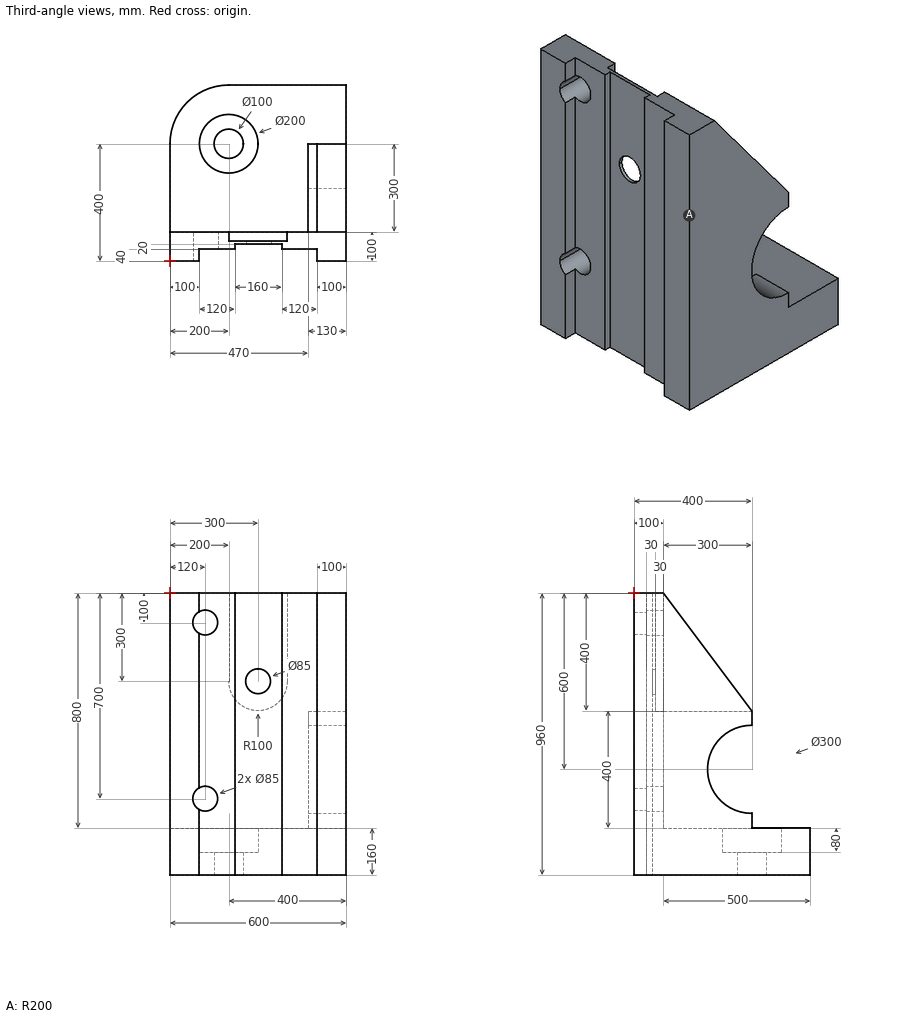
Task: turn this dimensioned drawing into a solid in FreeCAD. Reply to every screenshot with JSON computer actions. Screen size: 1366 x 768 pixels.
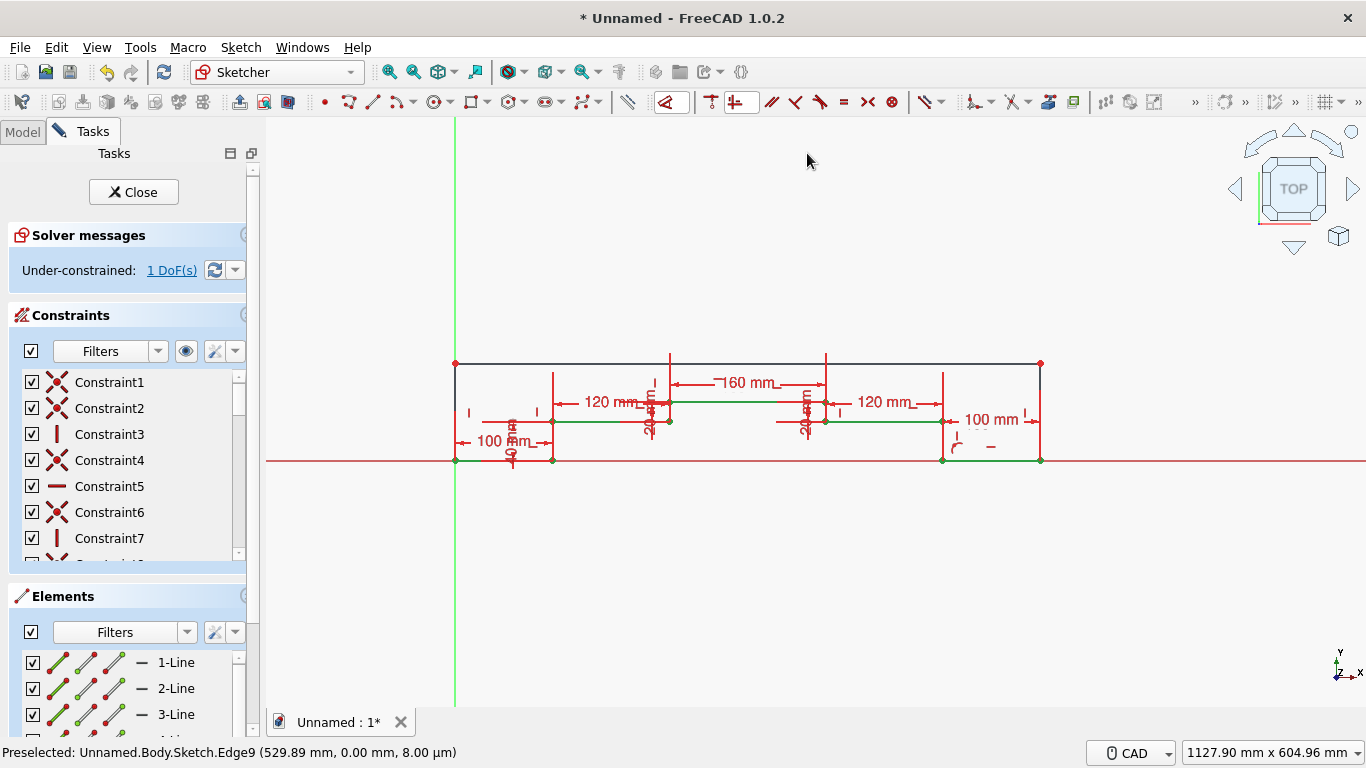
{"action": "left_click", "coordinate": [1040, 432]}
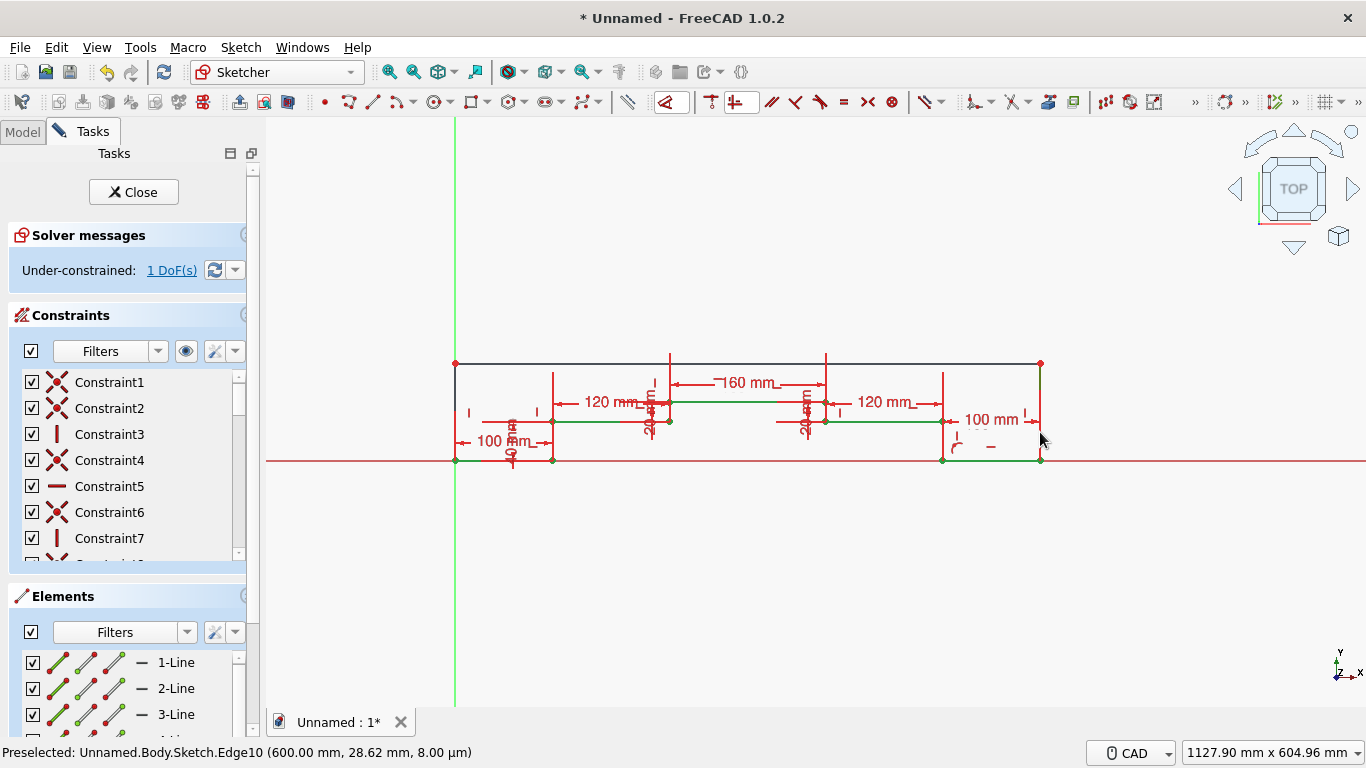
{"action": "key", "text": "i"}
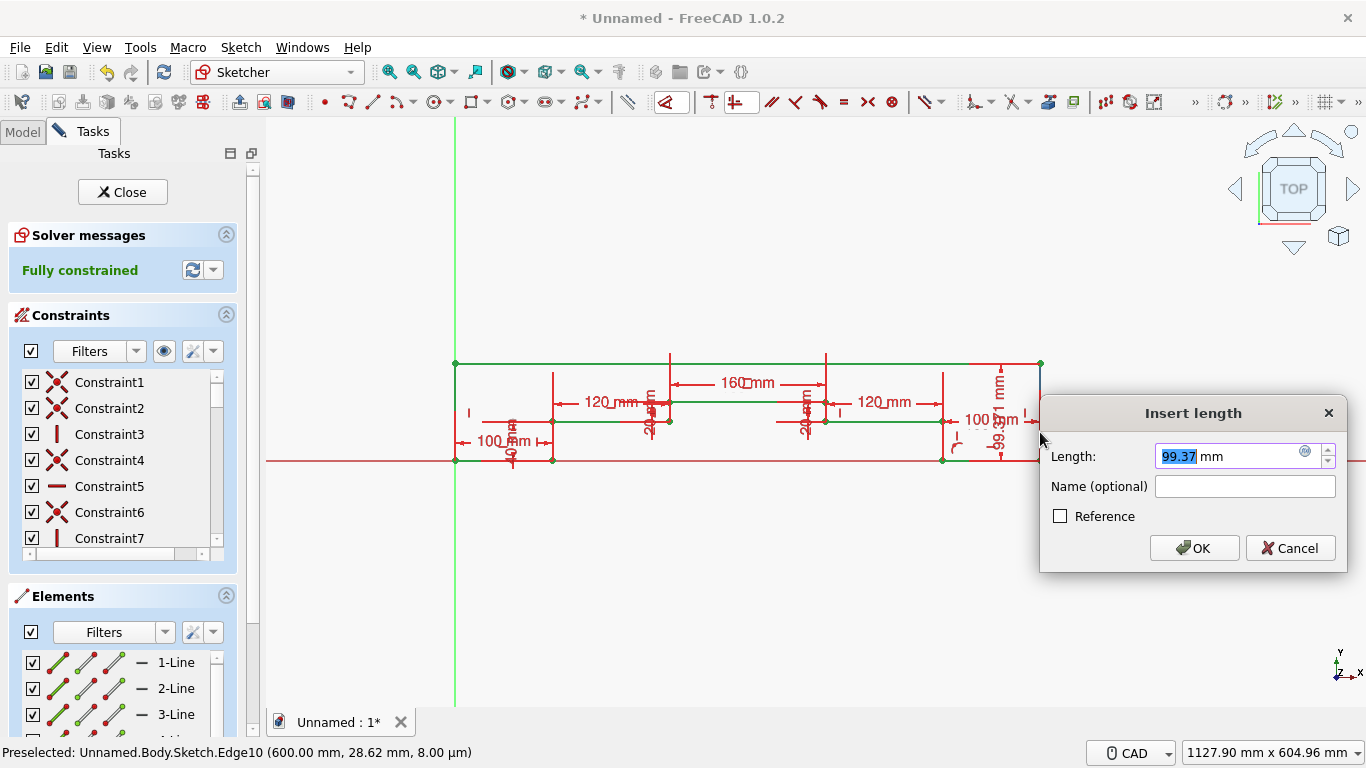
{"action": "type", "text": "100"}
{"action": "key", "text": "Return"}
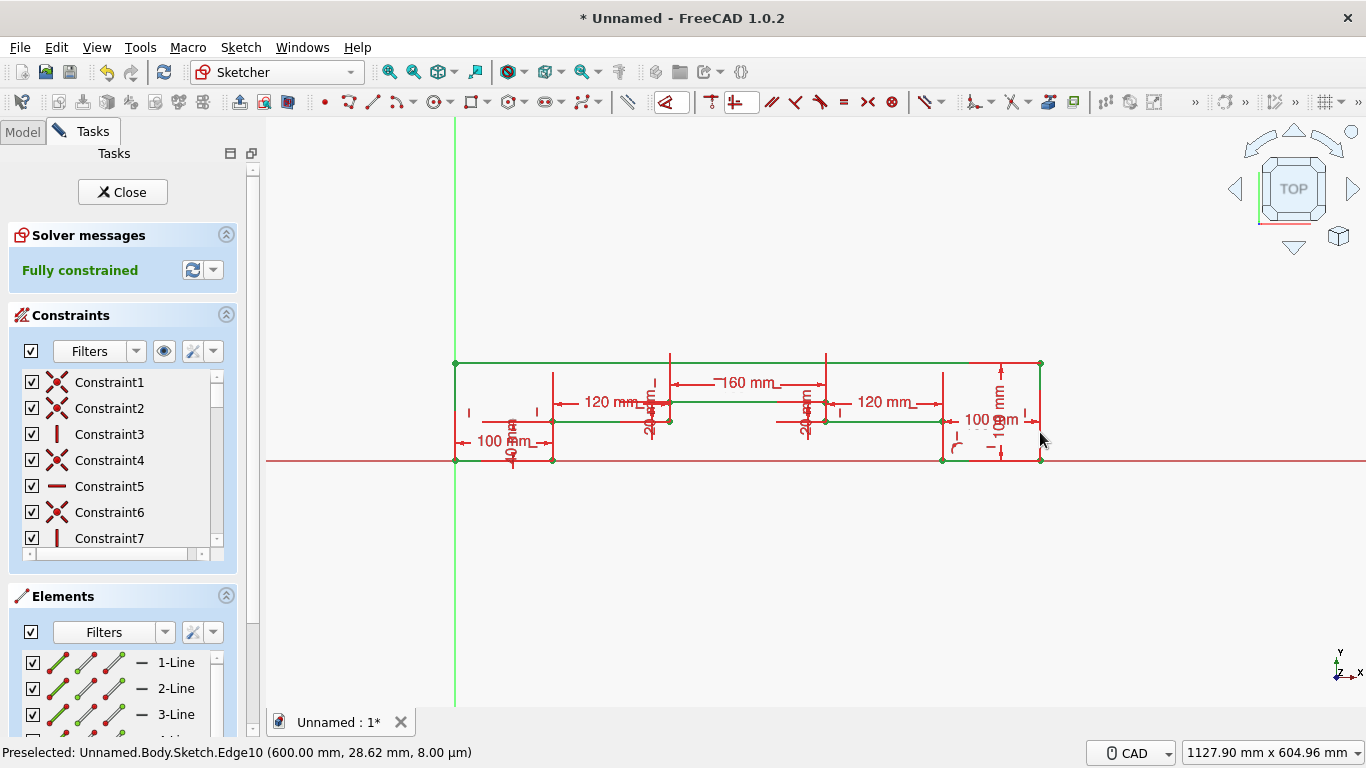
{"action": "left_click", "coordinate": [123, 192]}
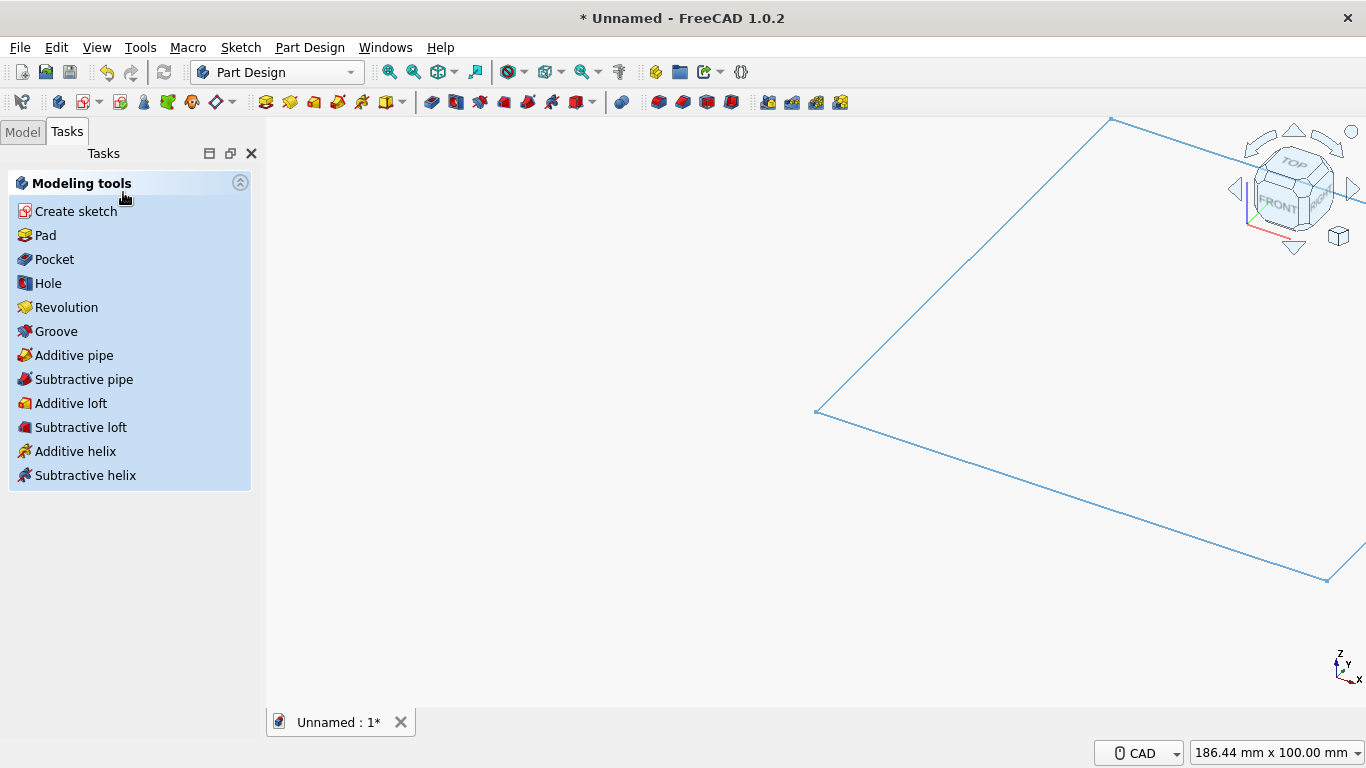
{"action": "left_click", "coordinate": [266, 102]}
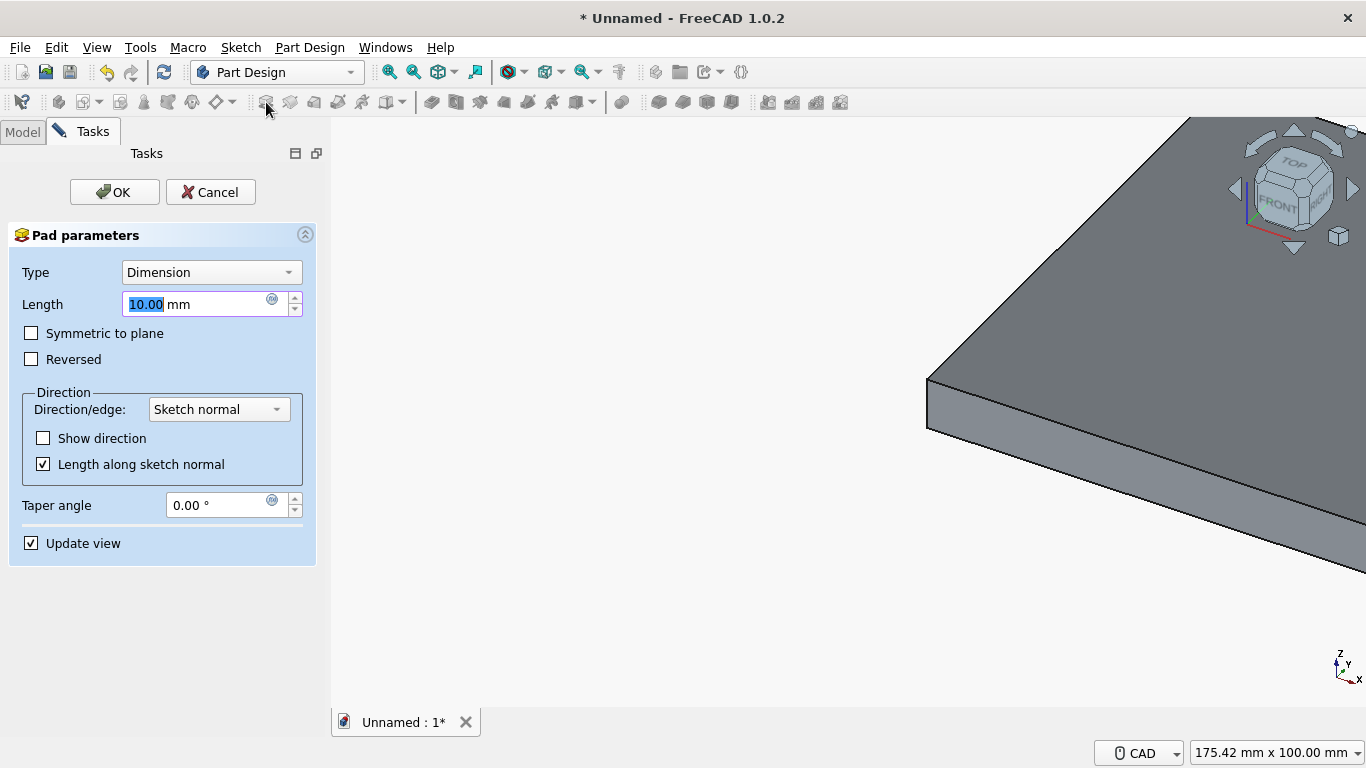
{"action": "type", "text": "960"}
{"action": "key", "text": "Tab"}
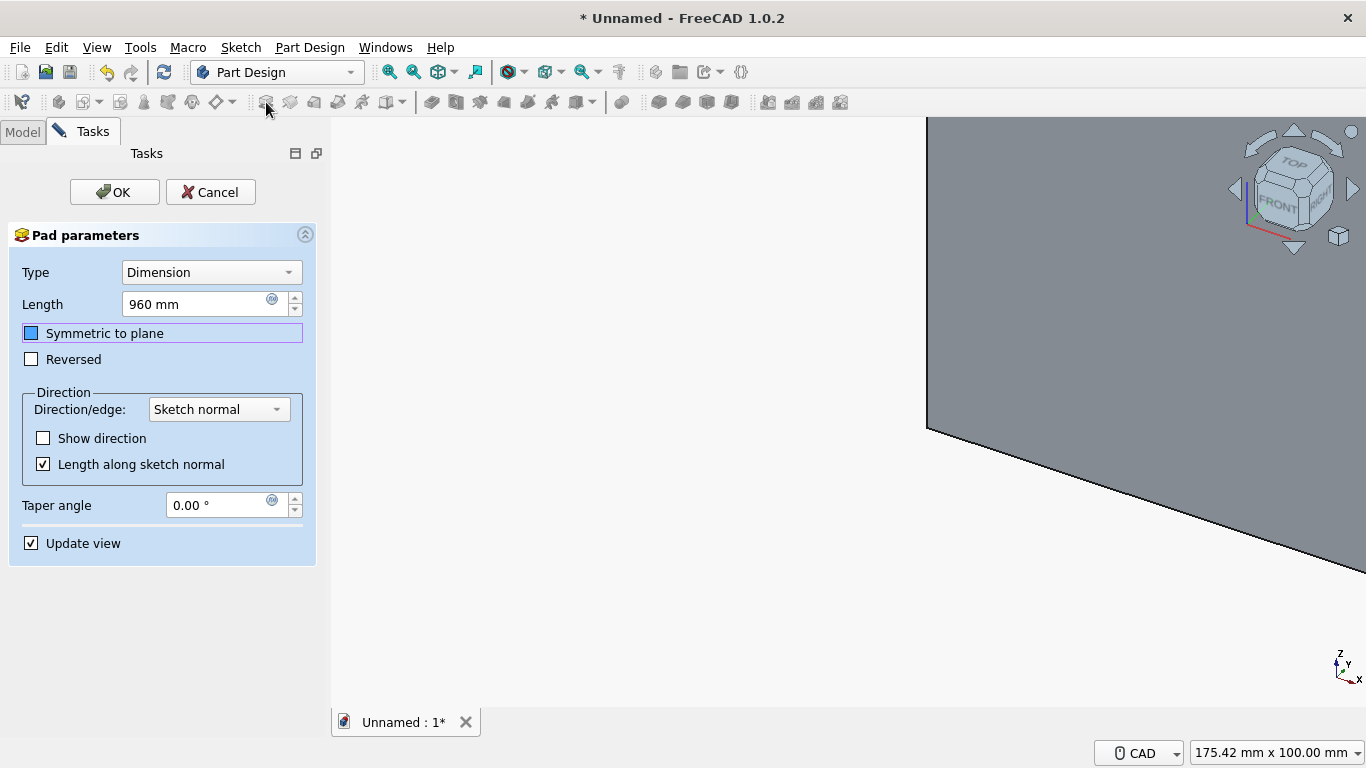
{"action": "left_click", "coordinate": [30, 359]}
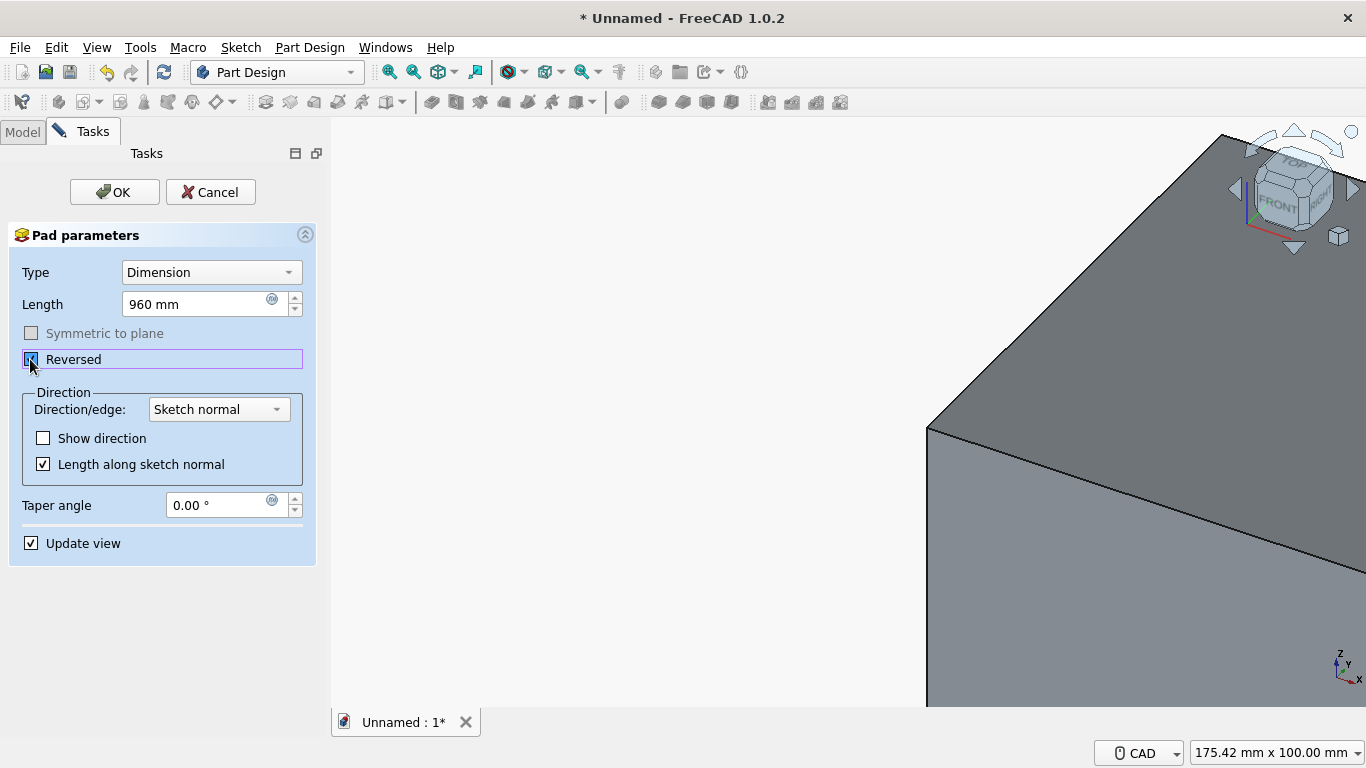
{"action": "left_click", "coordinate": [115, 192]}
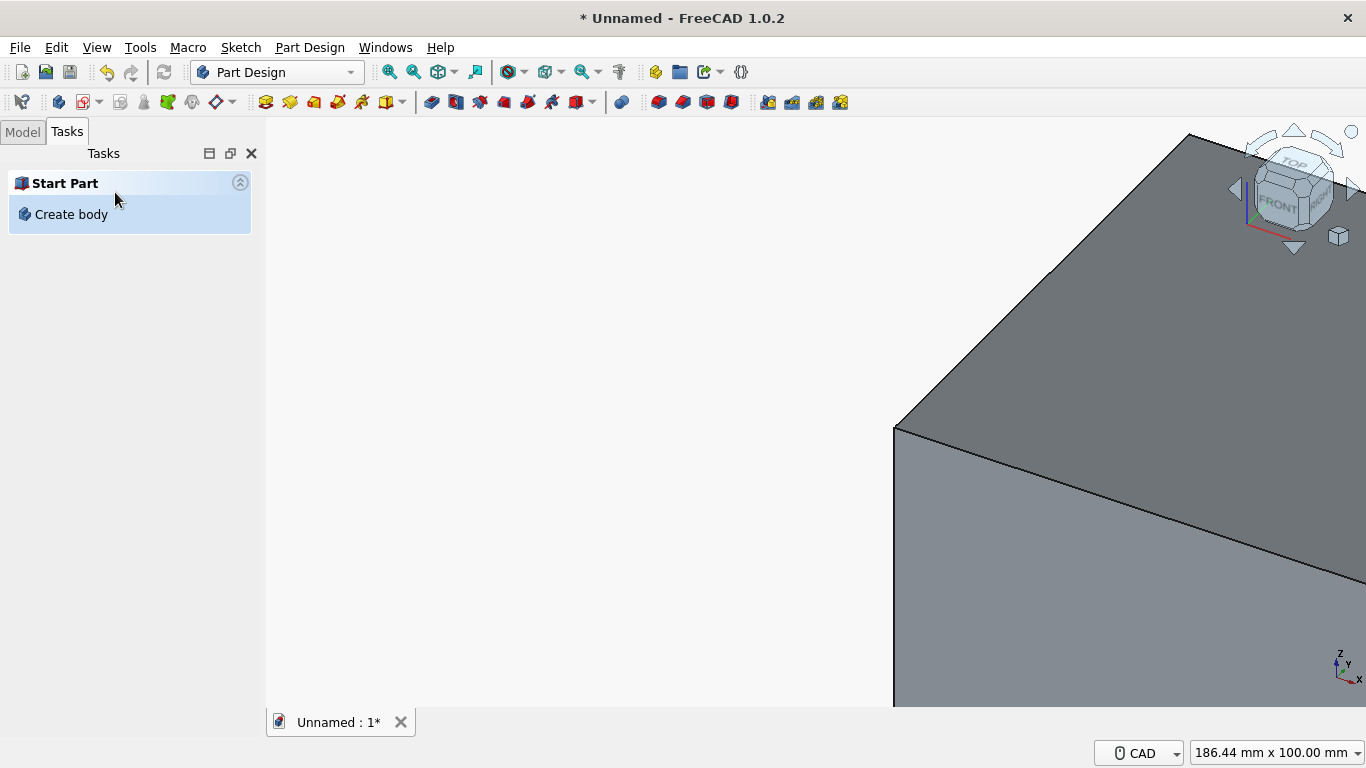
{"action": "left_click", "coordinate": [390, 72]}